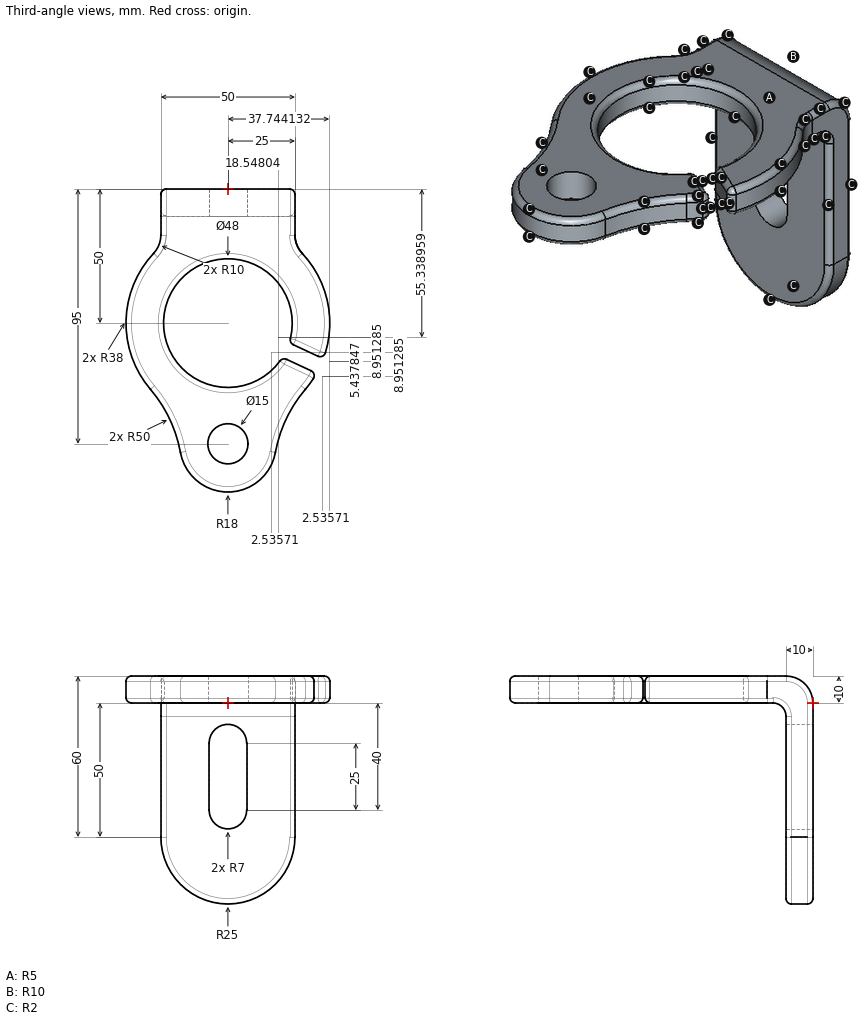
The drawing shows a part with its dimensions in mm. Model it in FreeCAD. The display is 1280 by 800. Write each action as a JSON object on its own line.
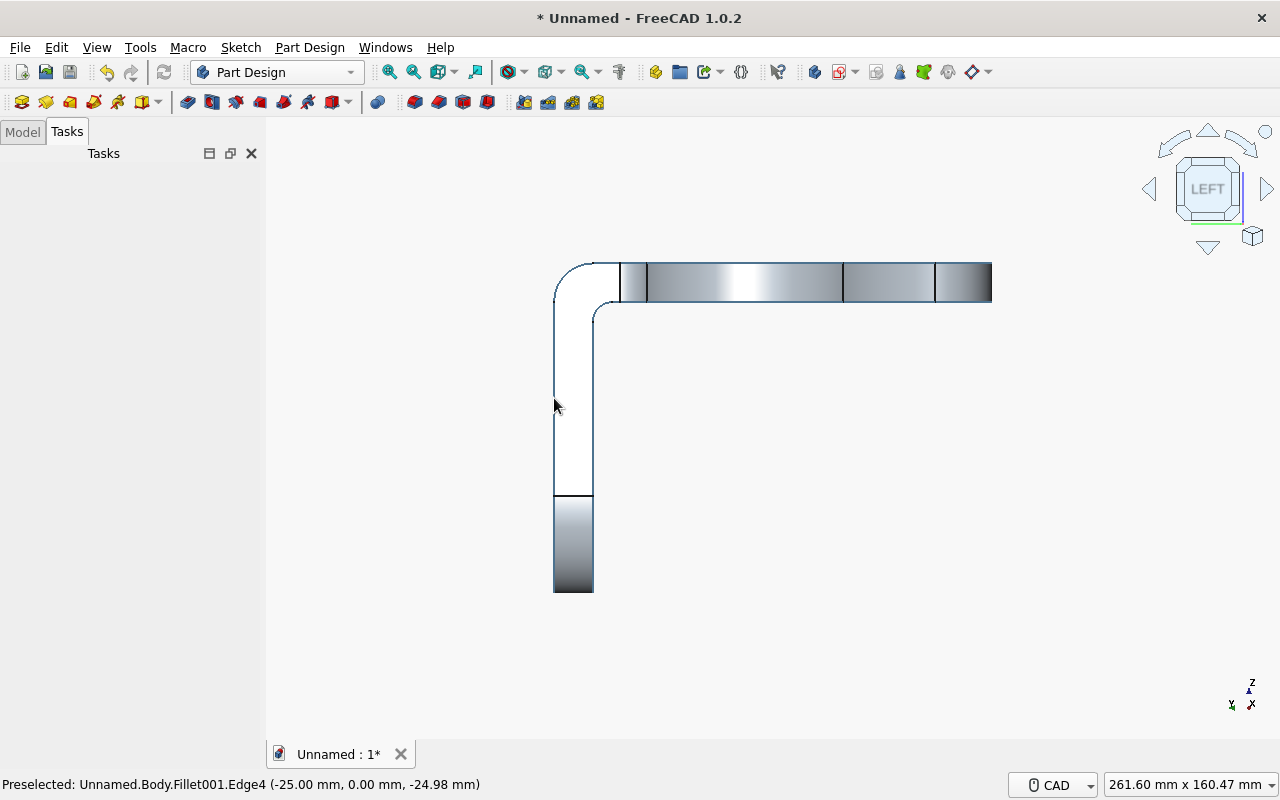
{"action": "left_click", "coordinate": [416, 102]}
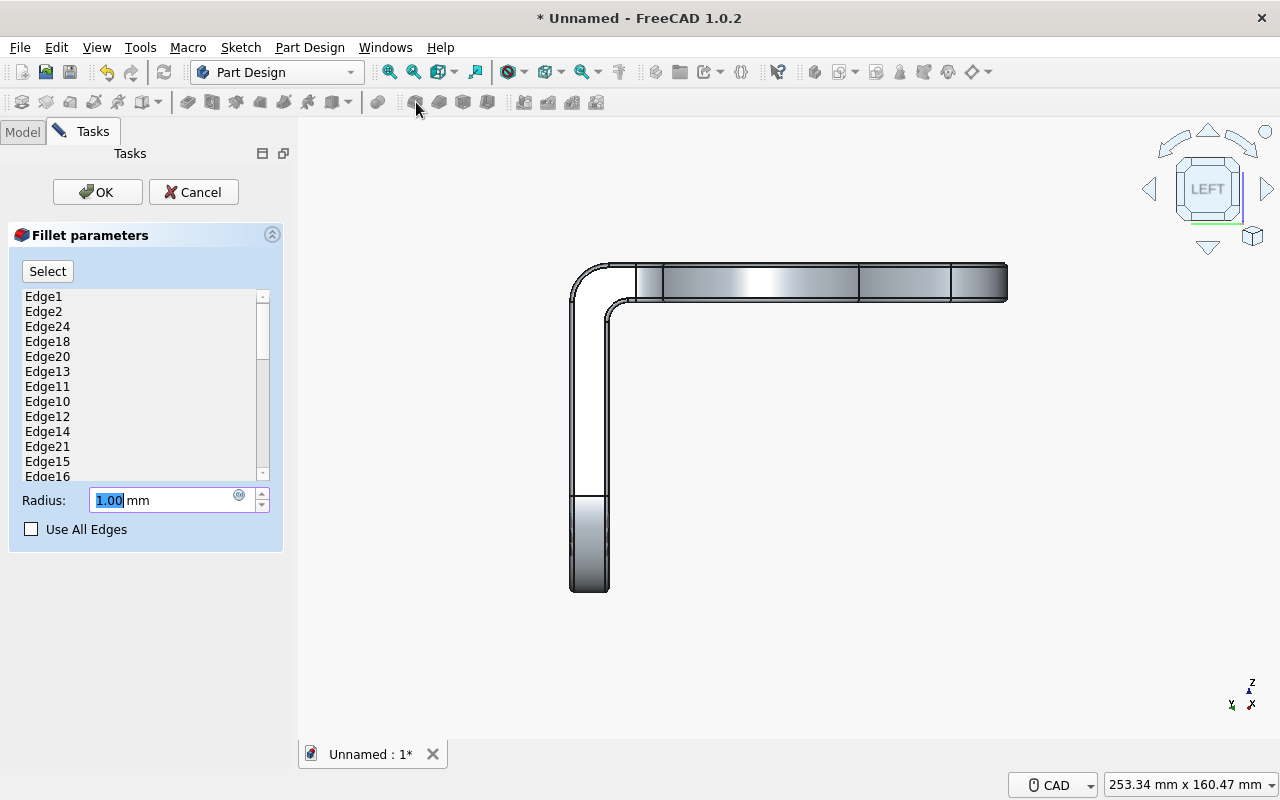
{"action": "type", "text": "2"}
{"action": "key", "text": "Tab"}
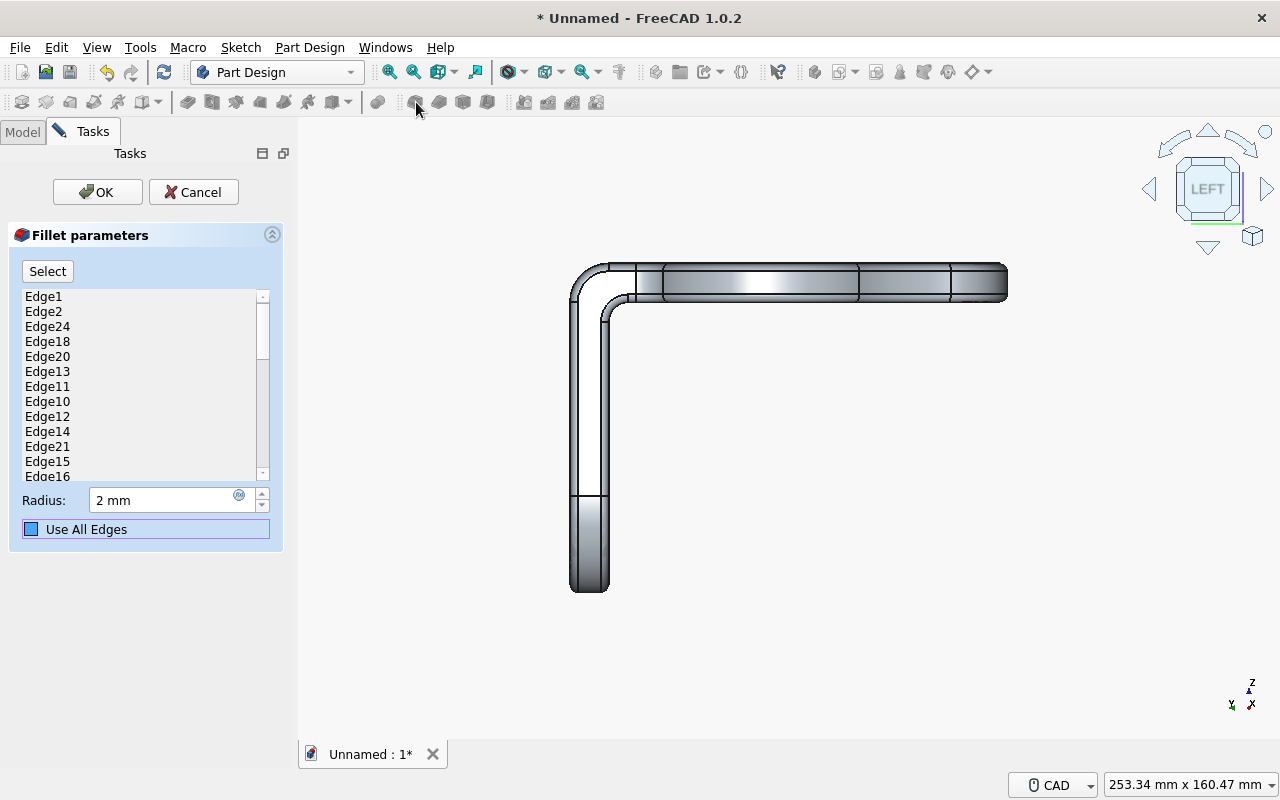
{"action": "left_click", "coordinate": [98, 192]}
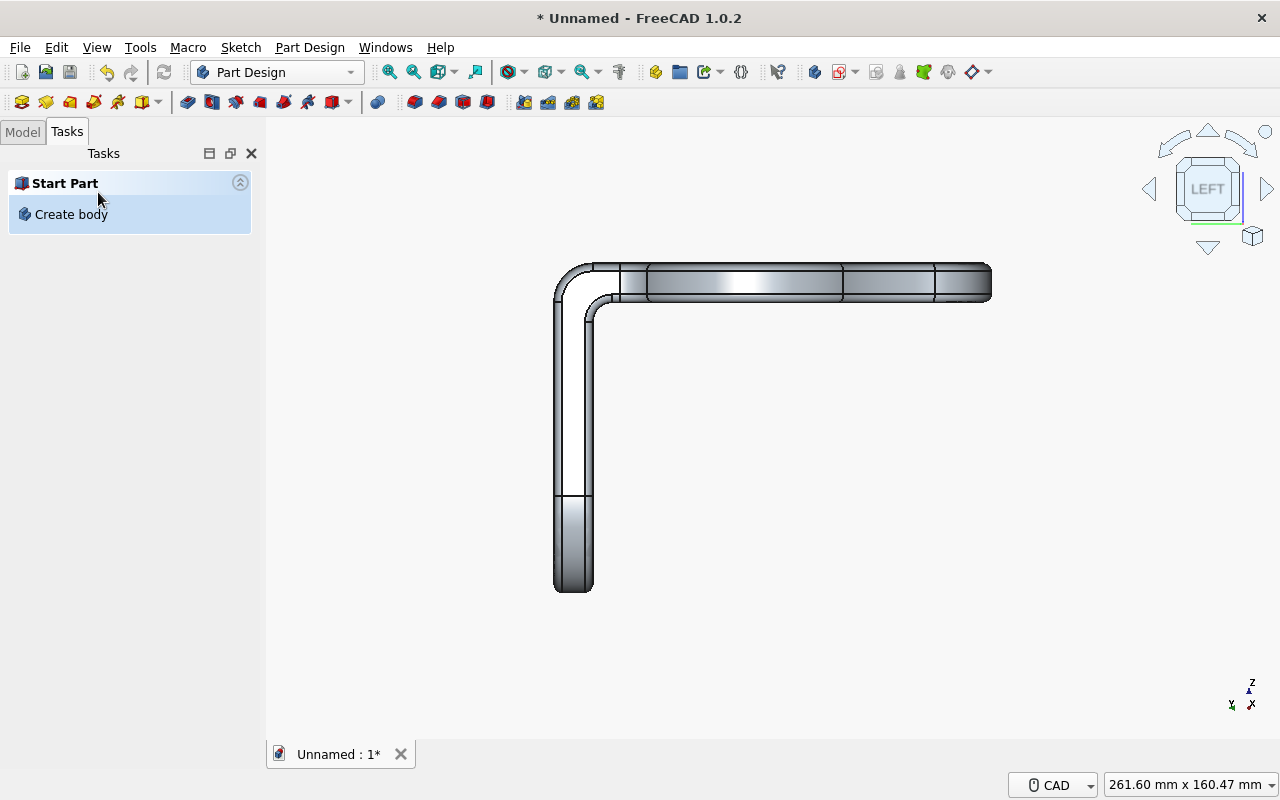
{"action": "key", "text": "0"}